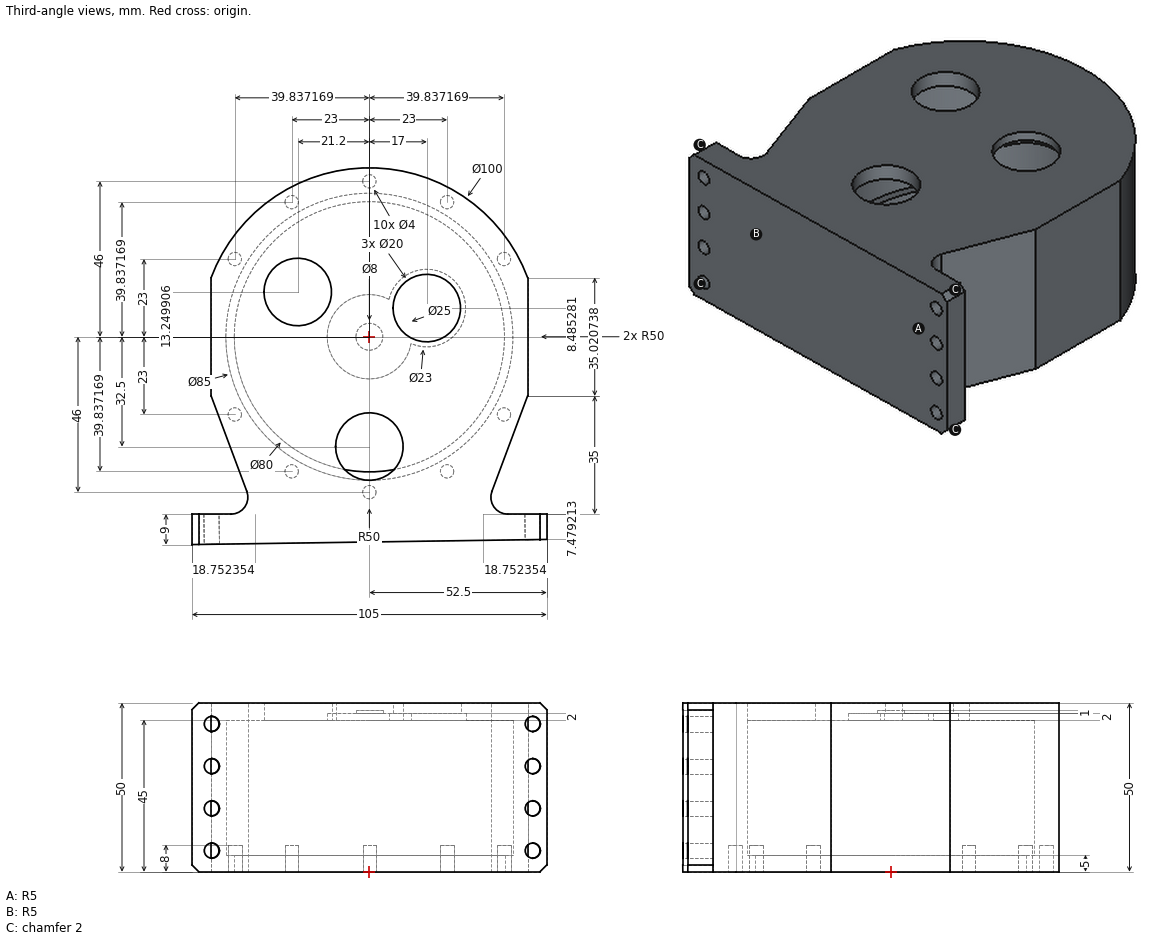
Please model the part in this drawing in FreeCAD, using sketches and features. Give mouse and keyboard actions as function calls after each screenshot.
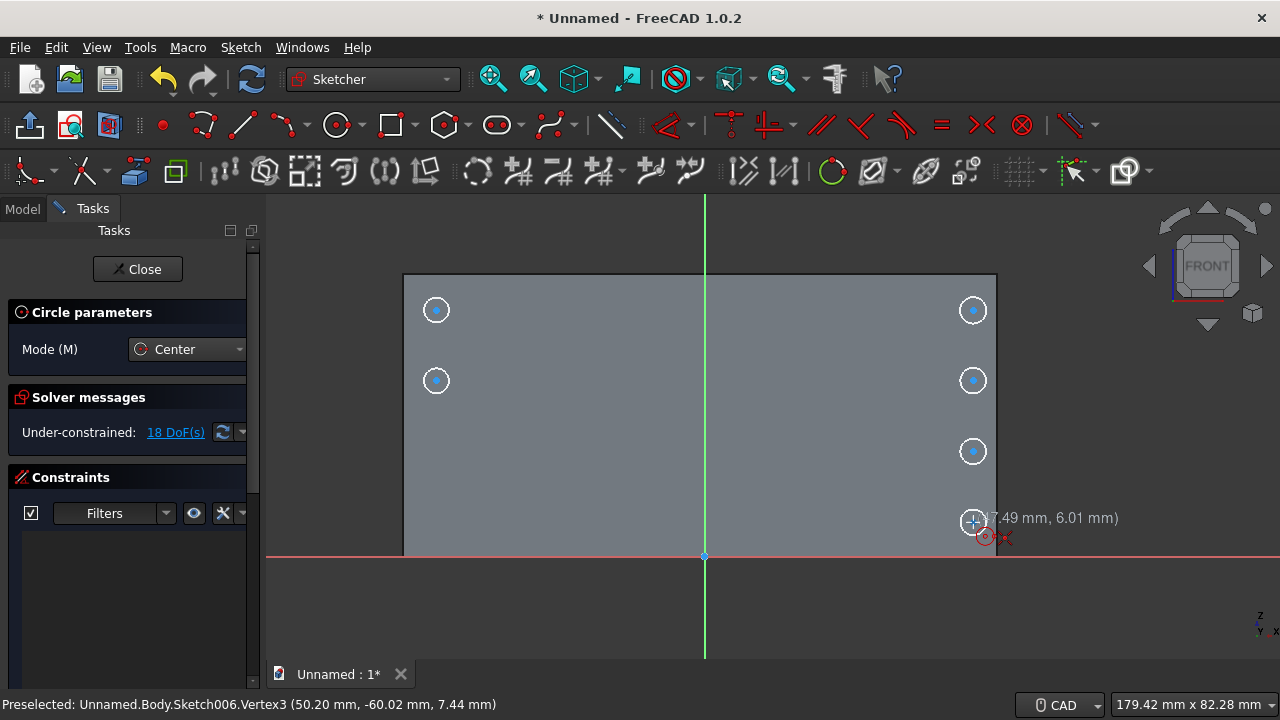
scroll(436, 451, up, 3)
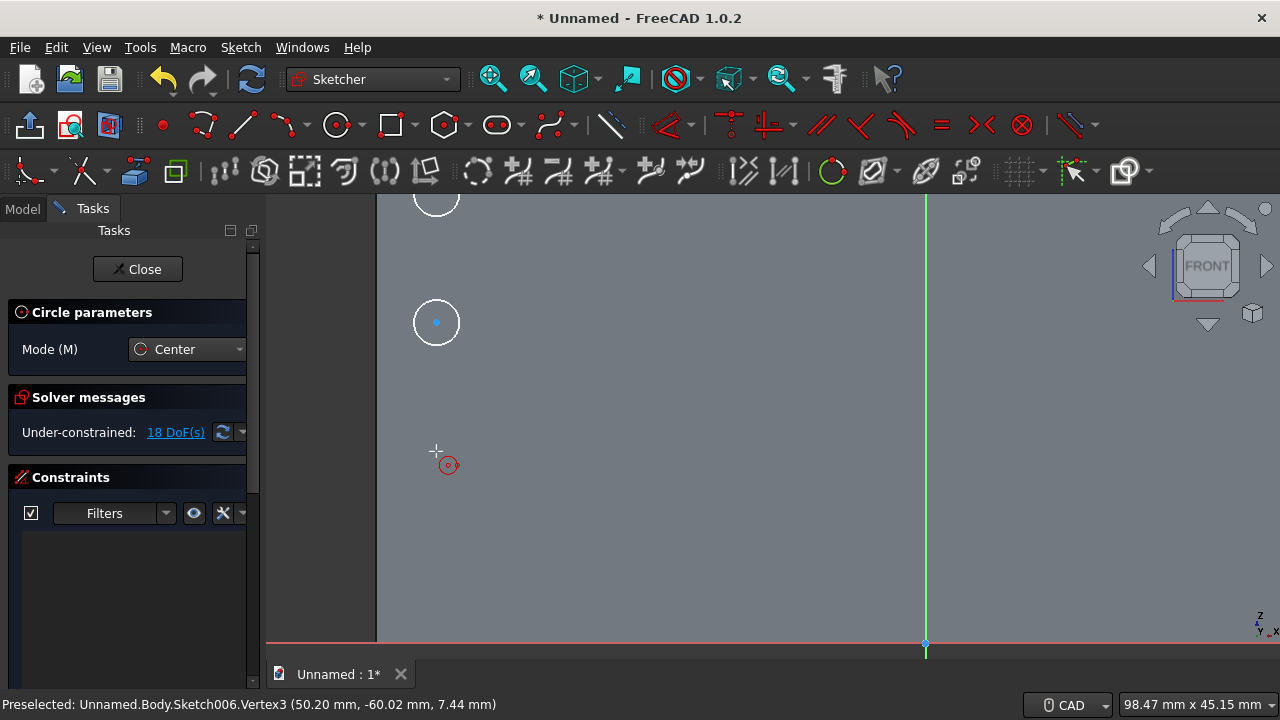
click(437, 450)
click(453, 434)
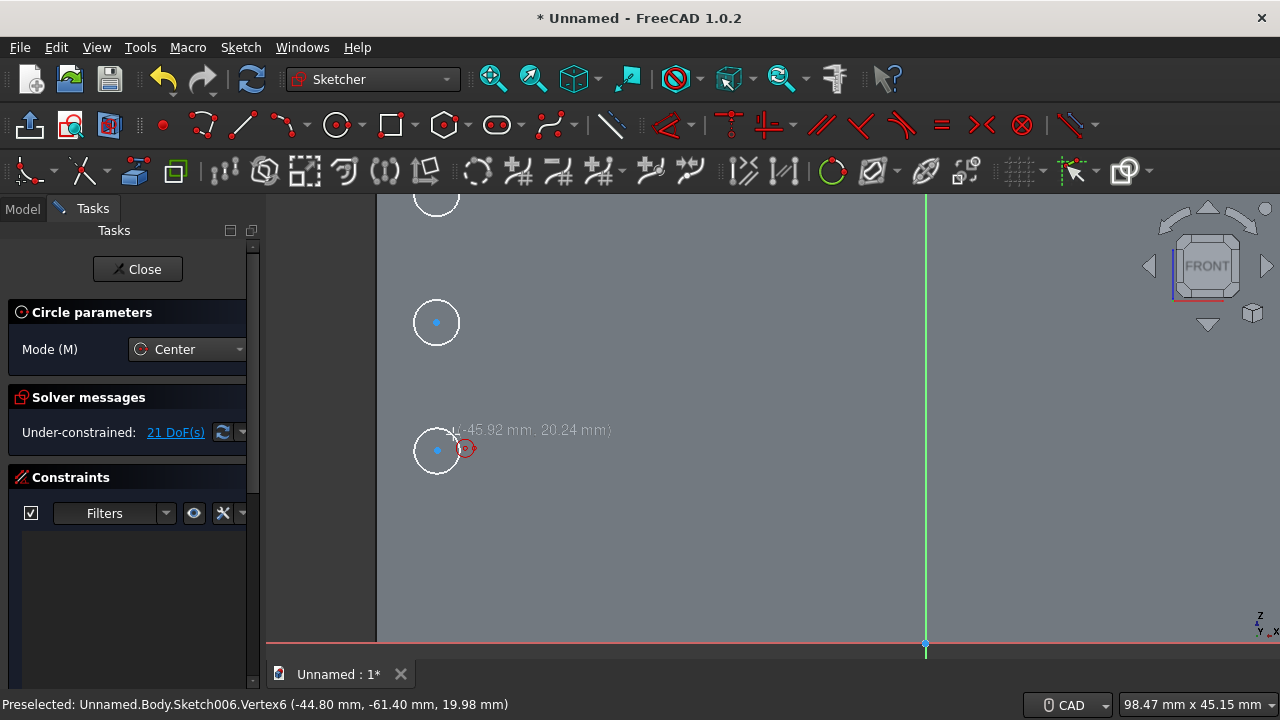
click(437, 579)
click(453, 563)
key(Escape)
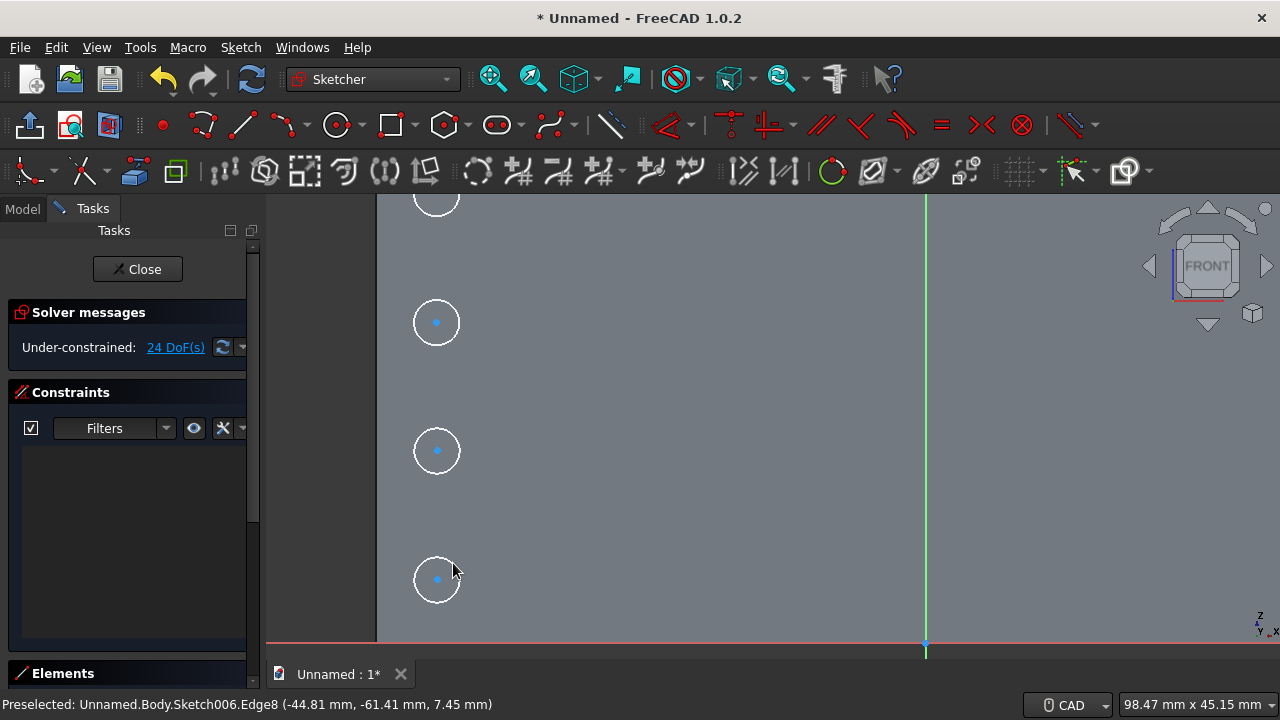
scroll(435, 451, down, 3)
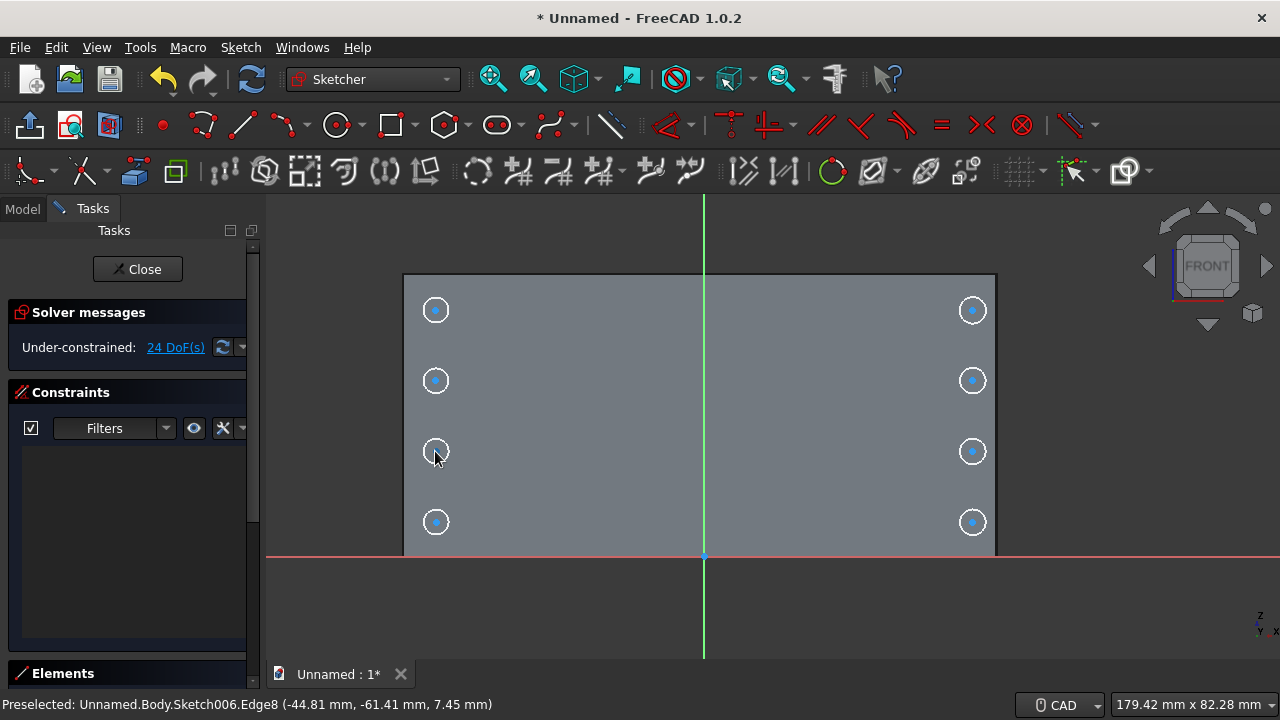
click(445, 301)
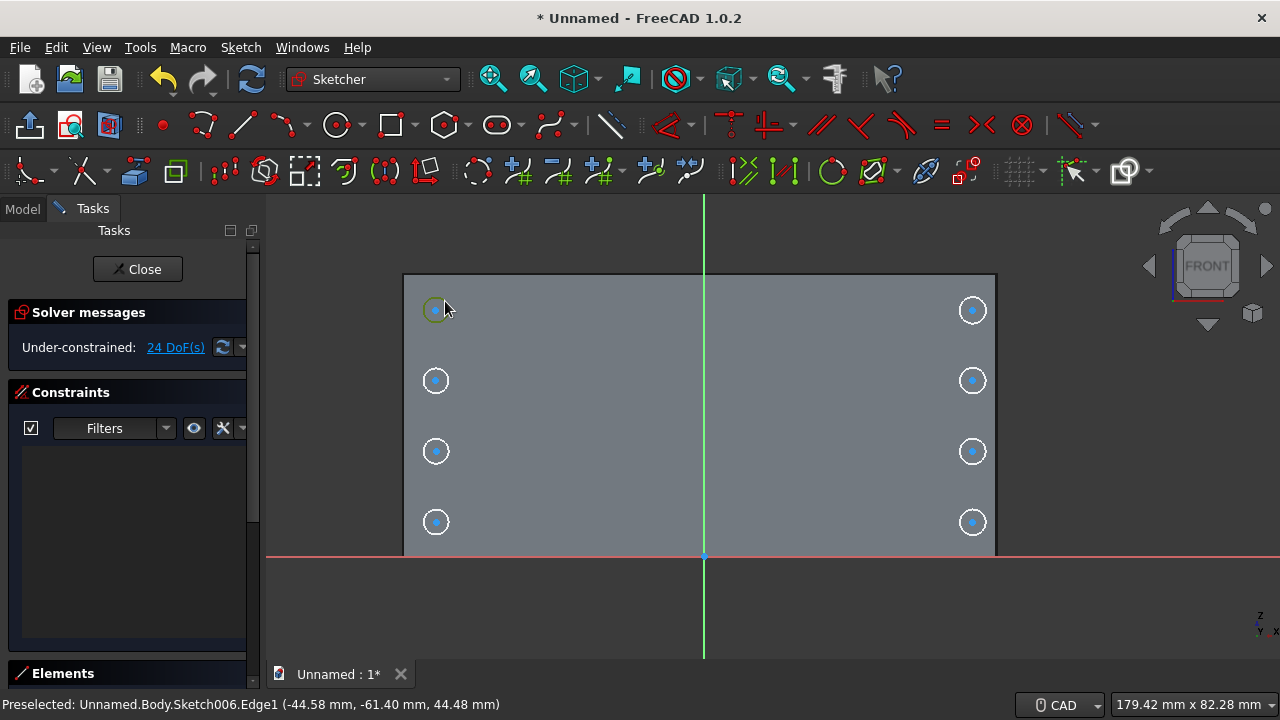
click(445, 372)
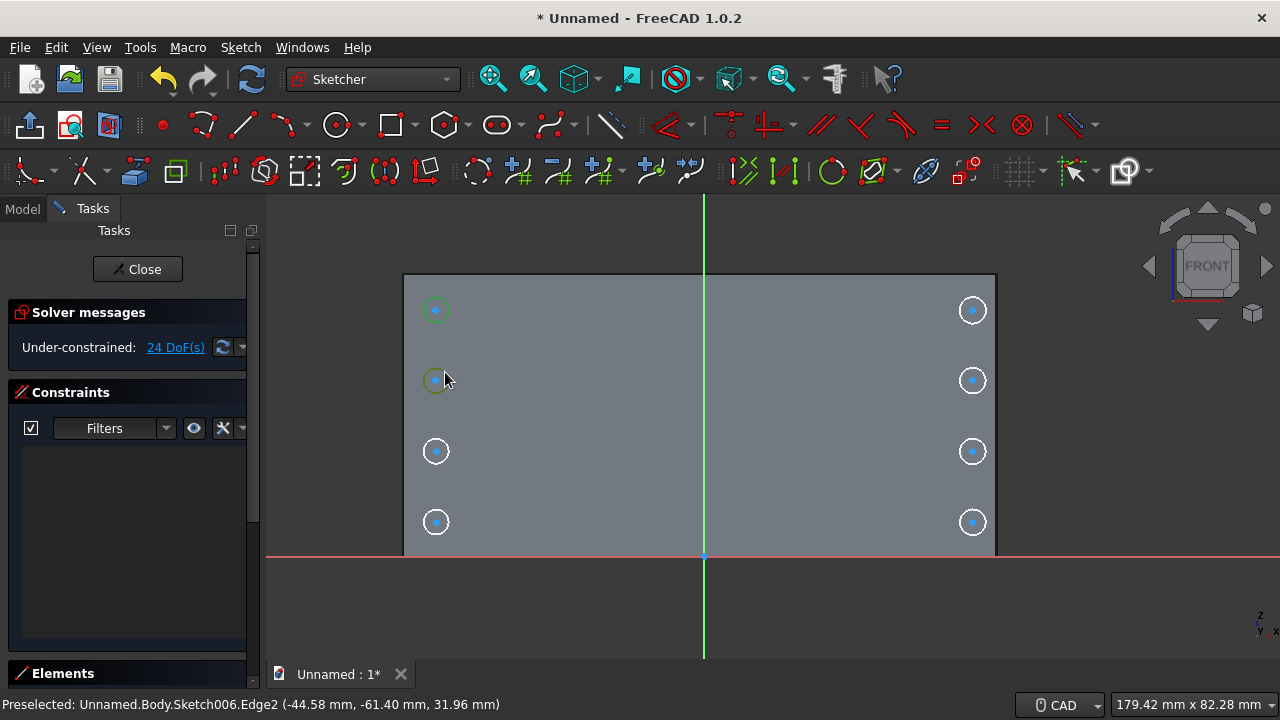
click(982, 372)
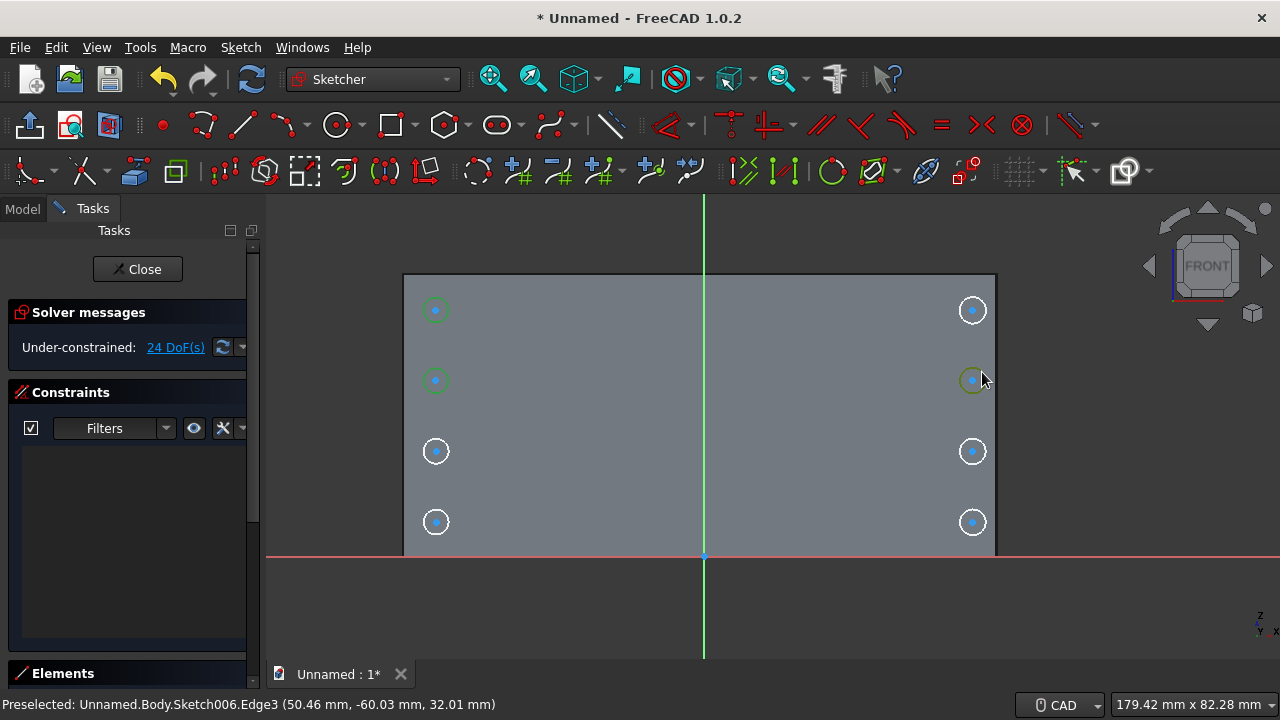
click(982, 301)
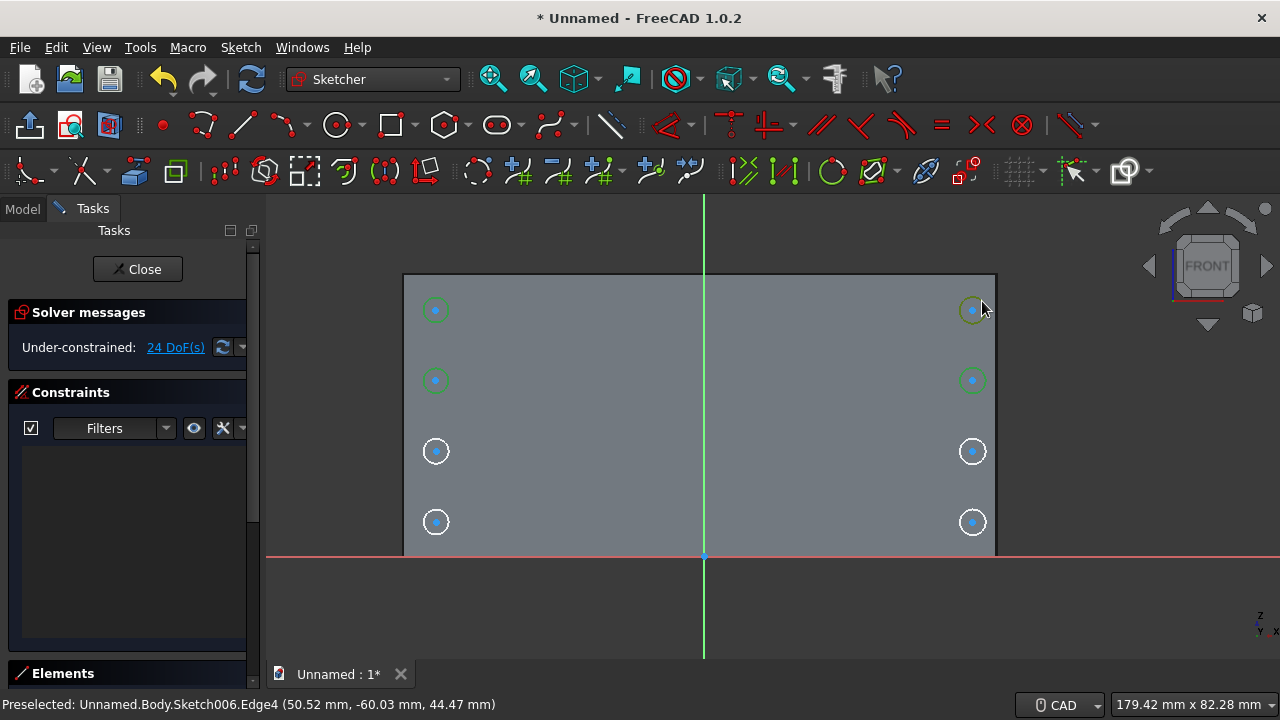
click(982, 442)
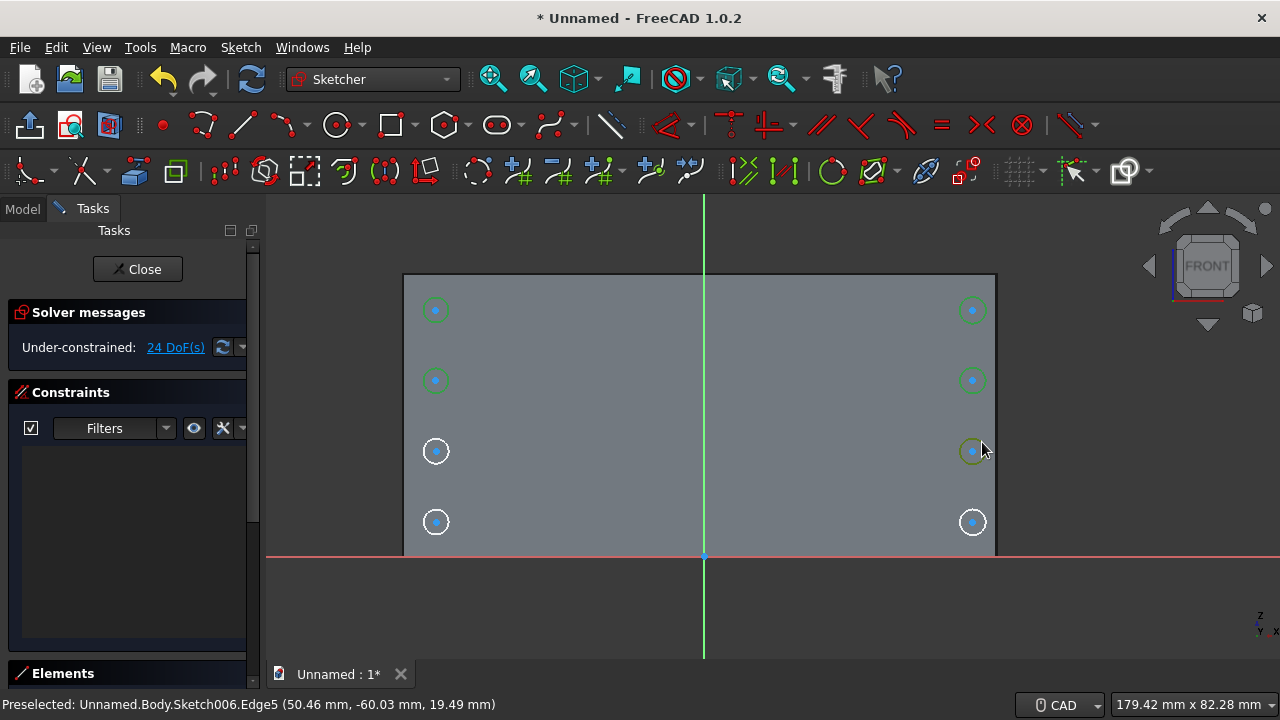
click(982, 513)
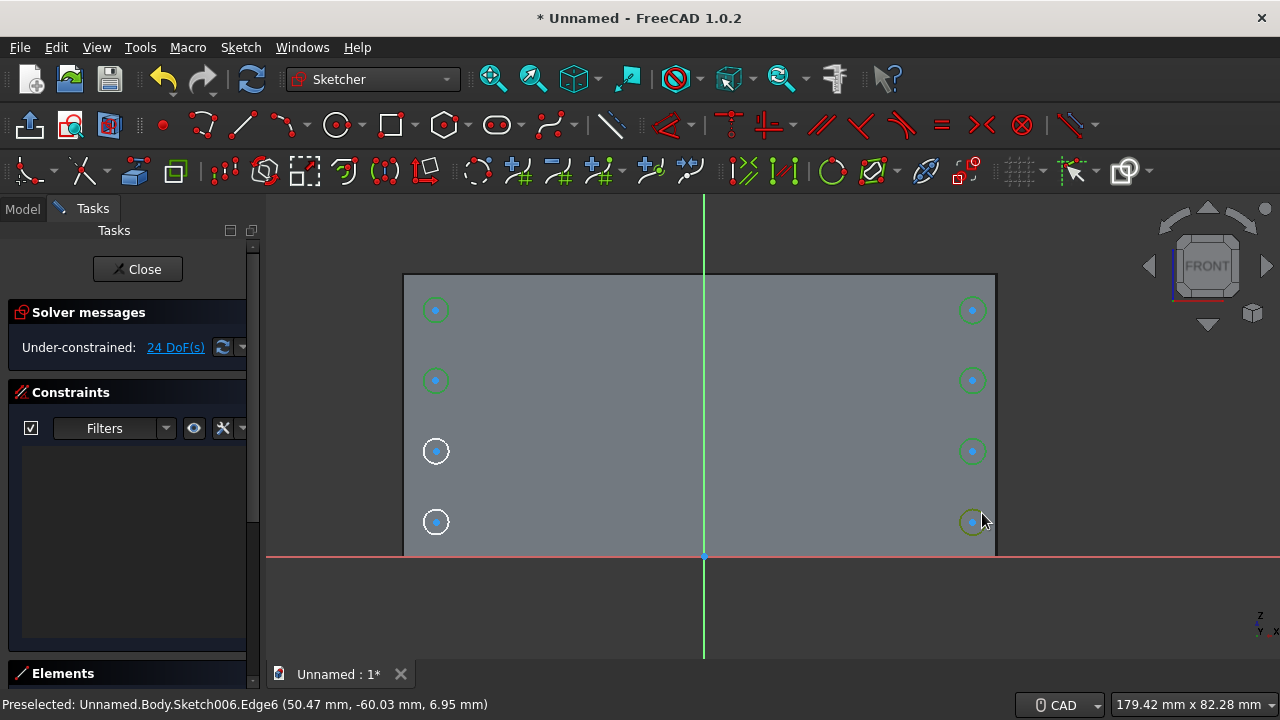
click(445, 442)